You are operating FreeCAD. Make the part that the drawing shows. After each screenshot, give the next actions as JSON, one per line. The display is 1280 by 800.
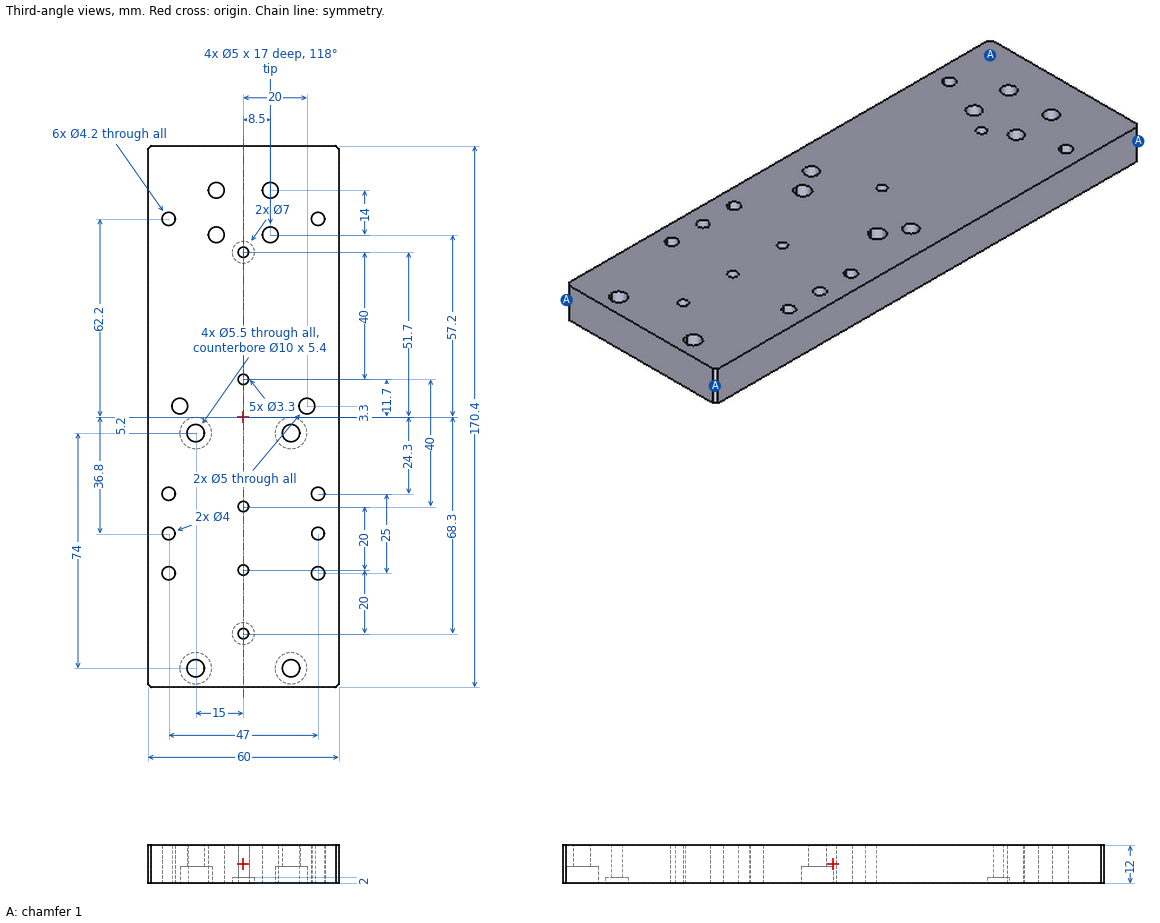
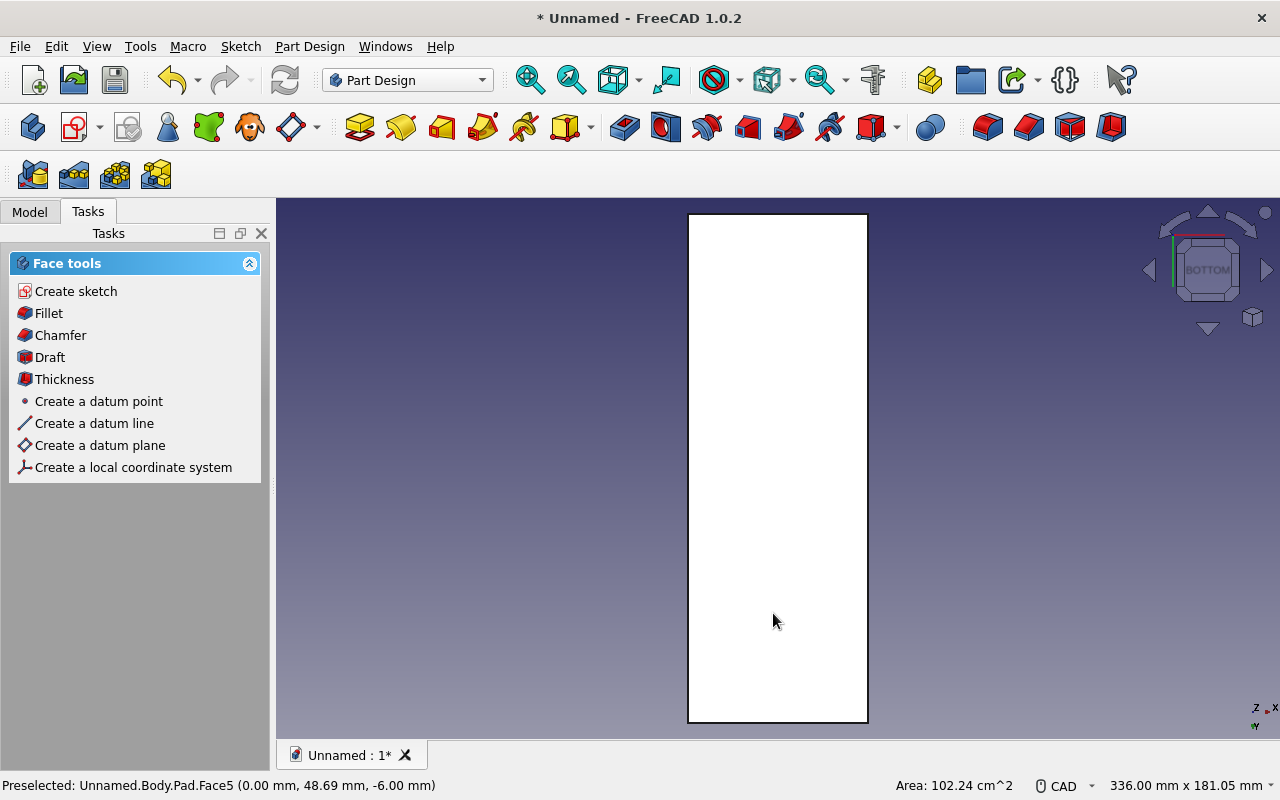
{"action": "left_click", "coordinate": [74, 128]}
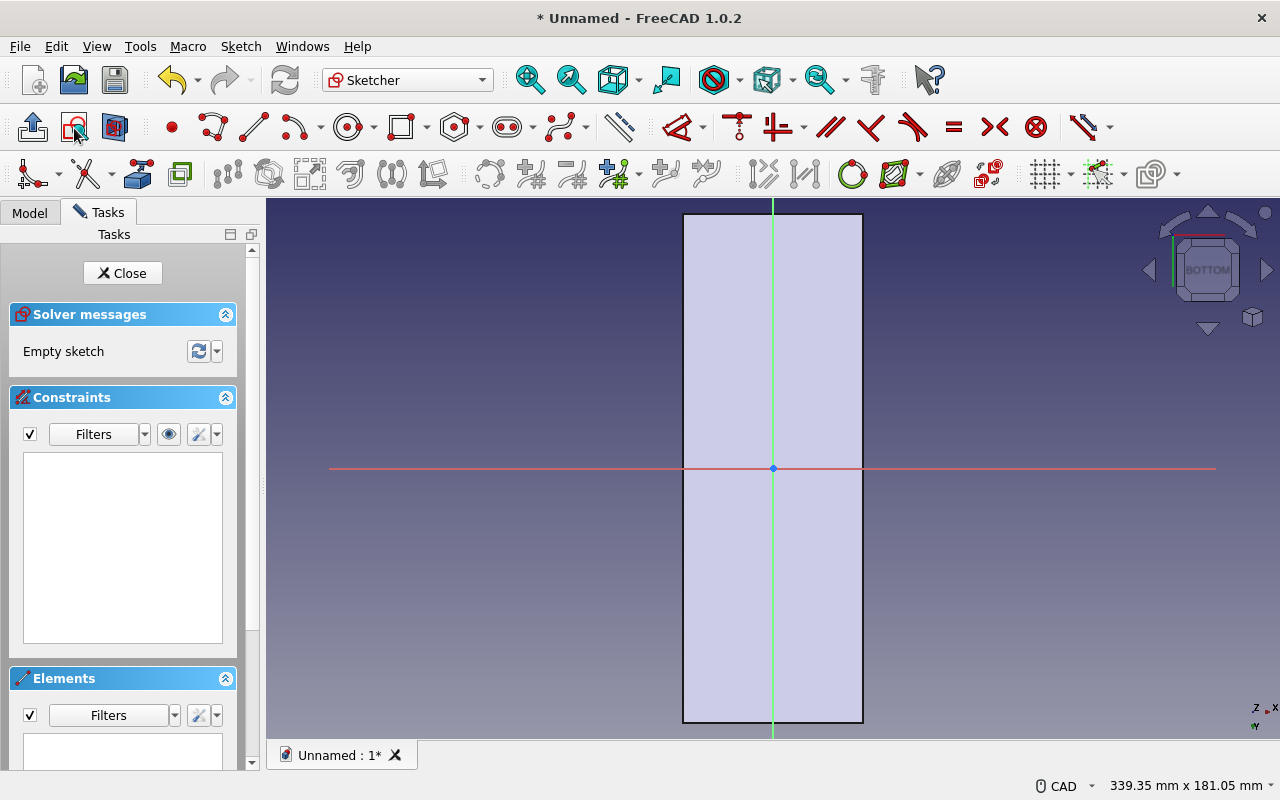
{"action": "scroll", "coordinate": [395, 711], "scroll_direction": "down", "scroll_amount": 1}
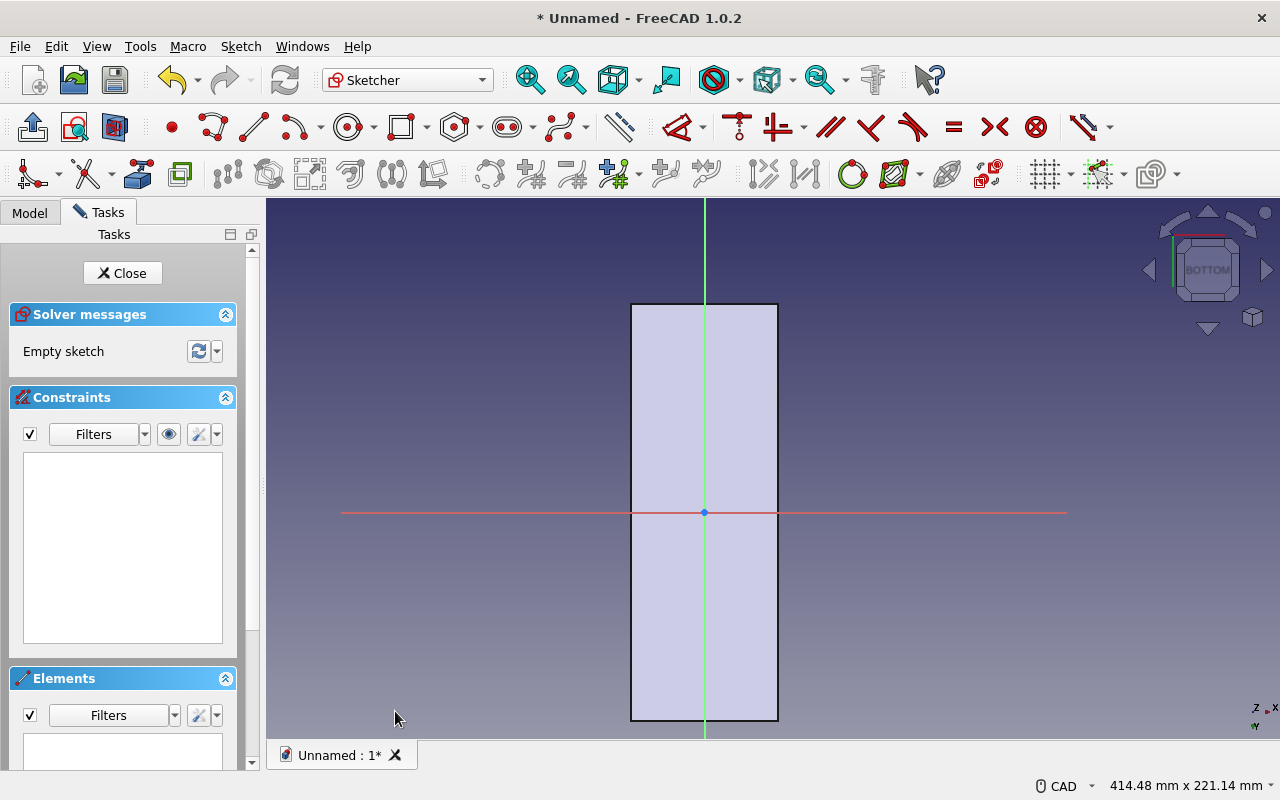
{"action": "scroll", "coordinate": [705, 344], "scroll_direction": "up", "scroll_amount": 3}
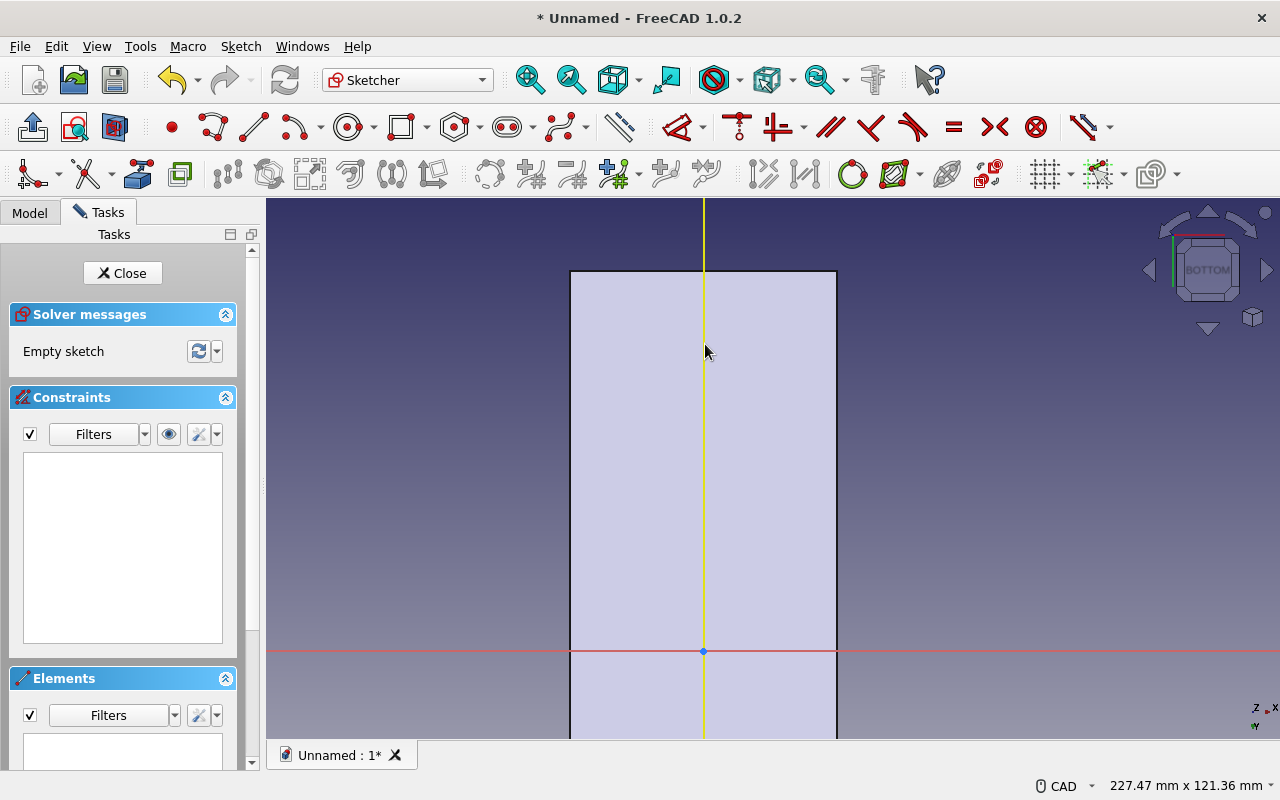
{"action": "left_click", "coordinate": [348, 128]}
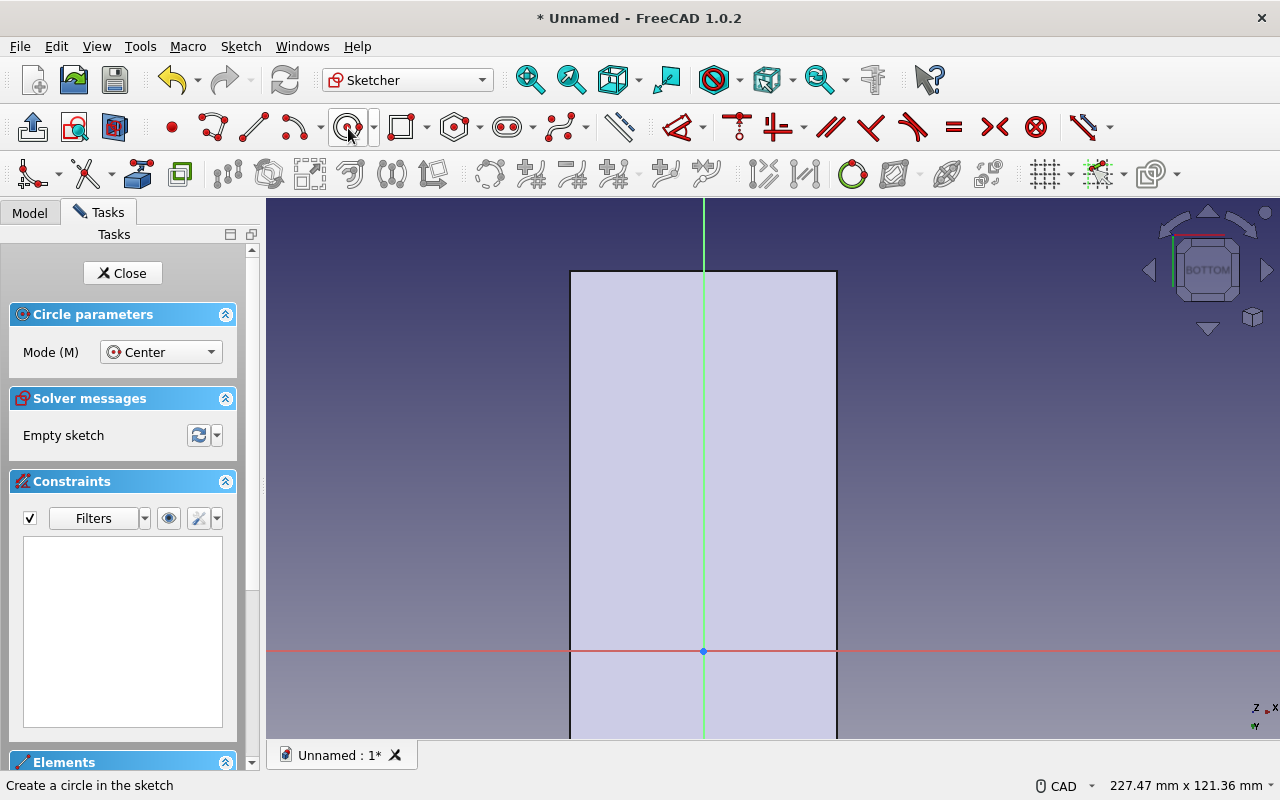
{"action": "scroll", "coordinate": [637, 628], "scroll_direction": "up", "scroll_amount": 4}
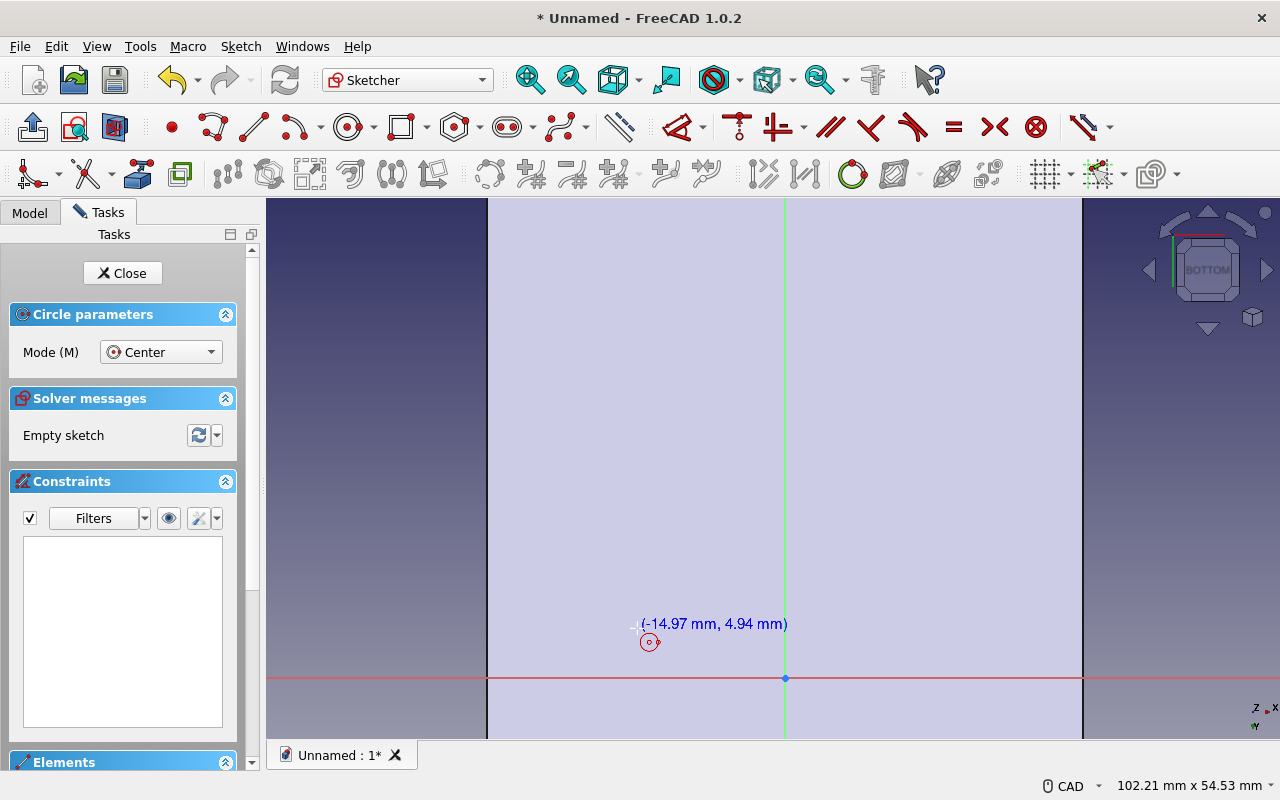
{"action": "left_click", "coordinate": [636, 627]}
{"action": "left_click", "coordinate": [656, 607]}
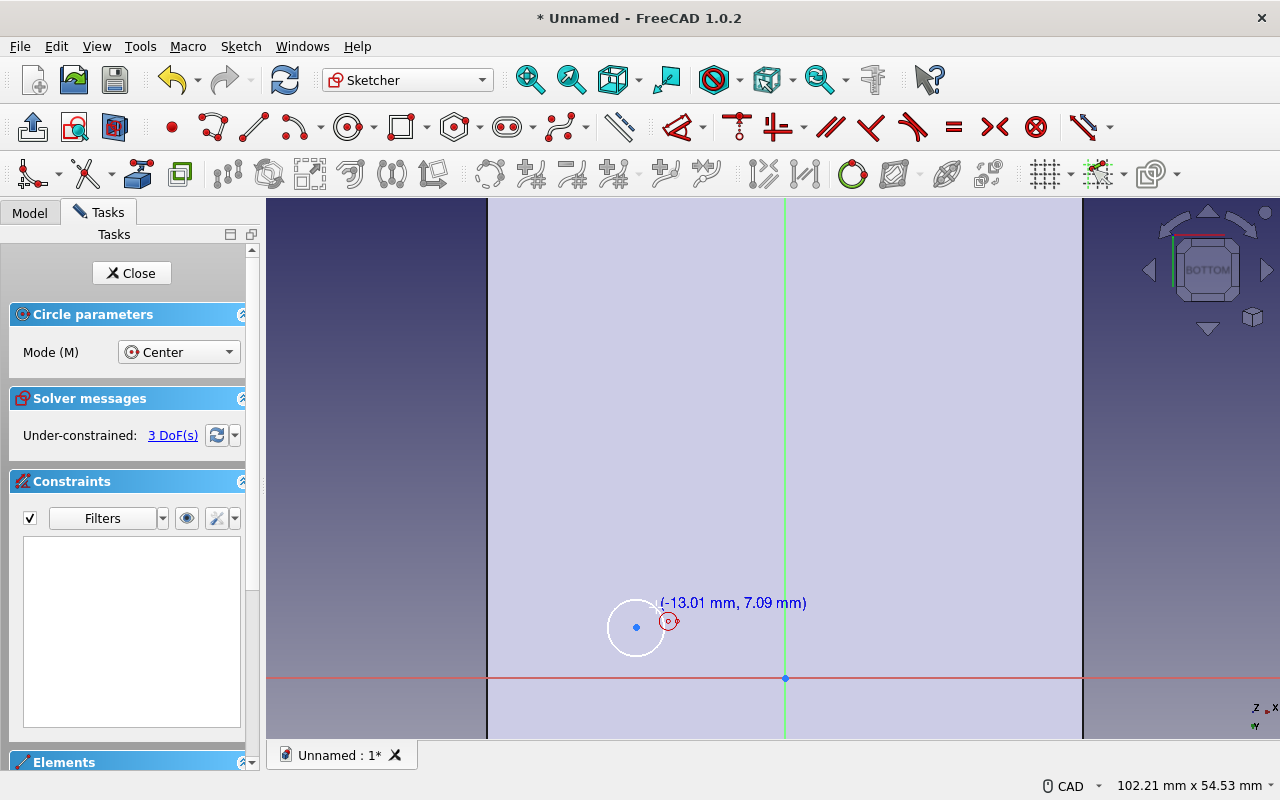
{"action": "left_click", "coordinate": [934, 627]}
{"action": "left_click", "coordinate": [953, 607]}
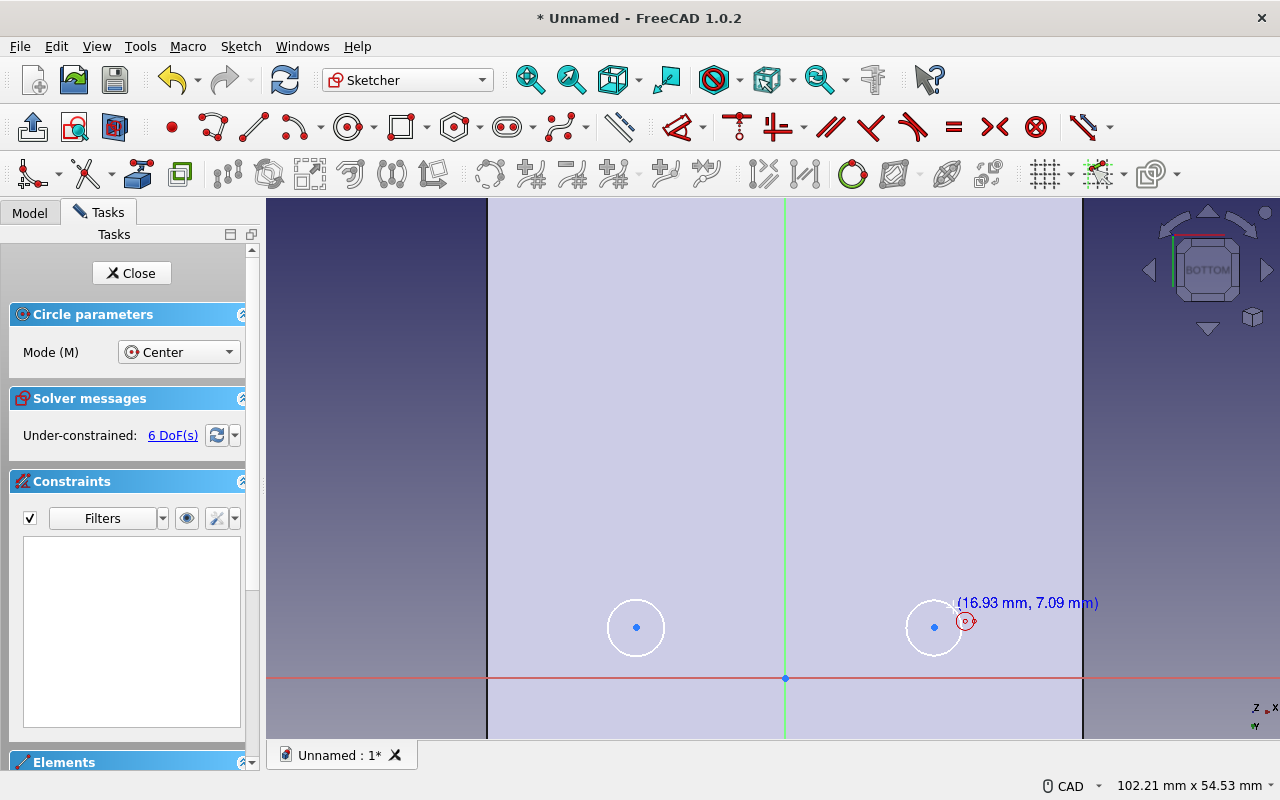
{"action": "scroll", "coordinate": [639, 629], "scroll_direction": "down", "scroll_amount": 4}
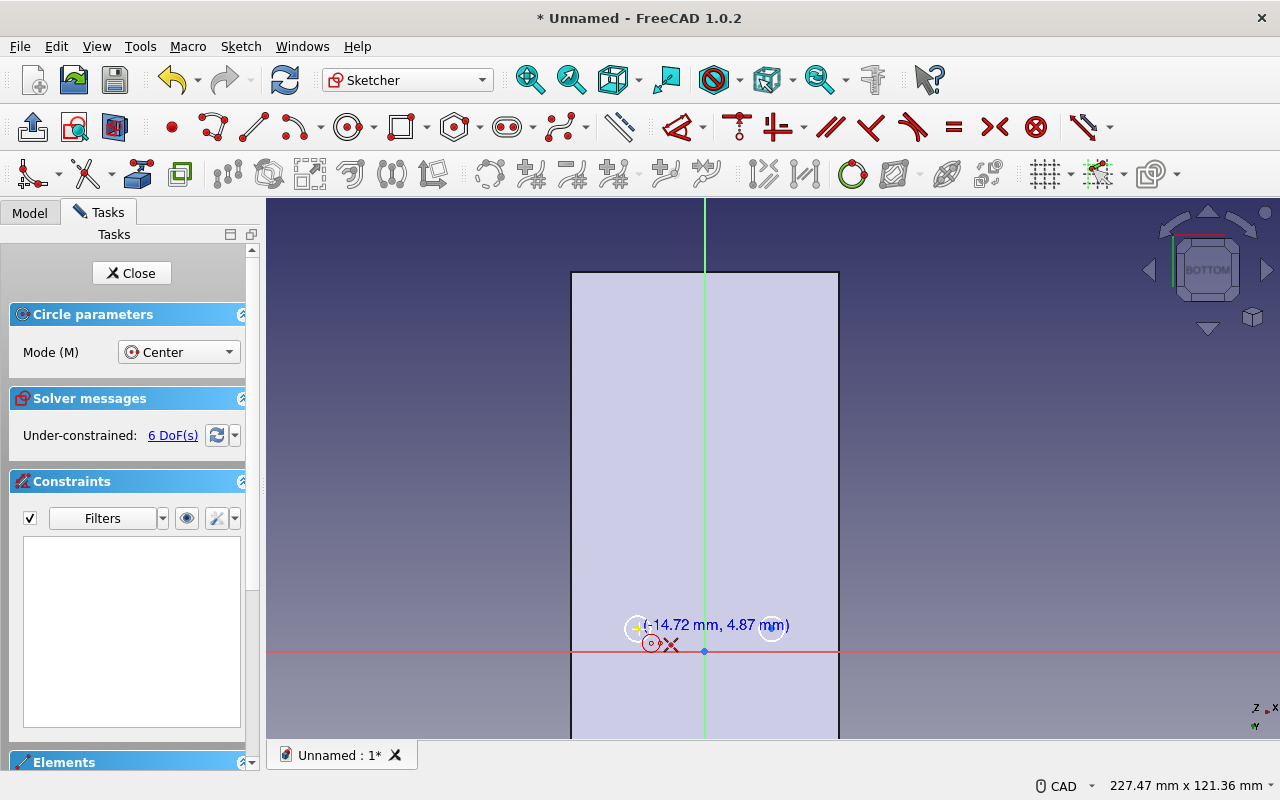
{"action": "scroll", "coordinate": [638, 299], "scroll_direction": "up", "scroll_amount": 4}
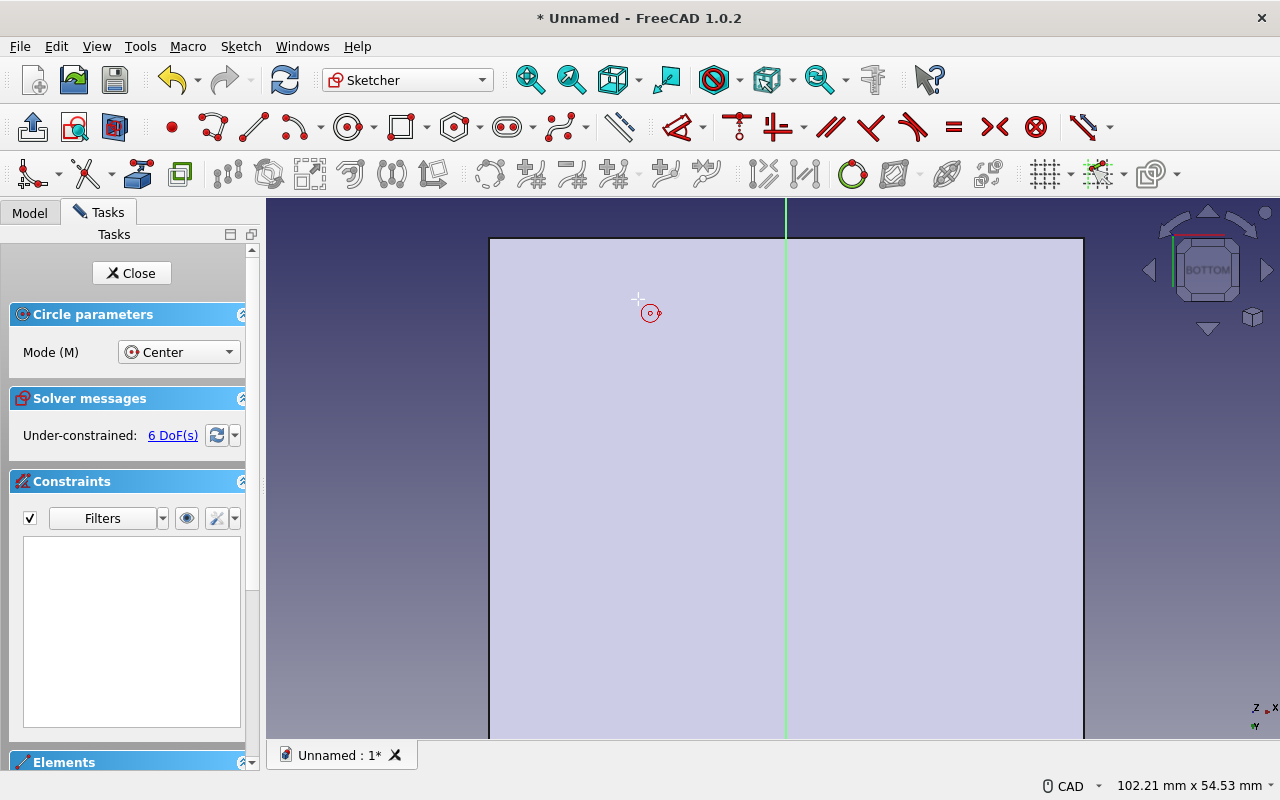
{"action": "left_click", "coordinate": [637, 298]}
{"action": "left_click", "coordinate": [657, 278]}